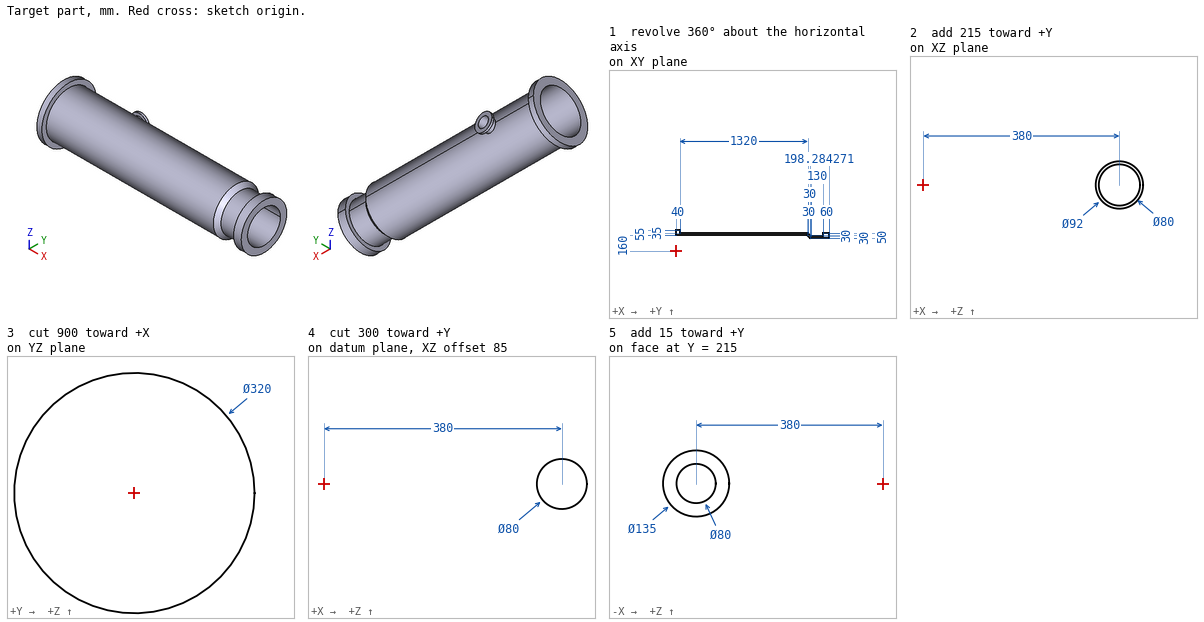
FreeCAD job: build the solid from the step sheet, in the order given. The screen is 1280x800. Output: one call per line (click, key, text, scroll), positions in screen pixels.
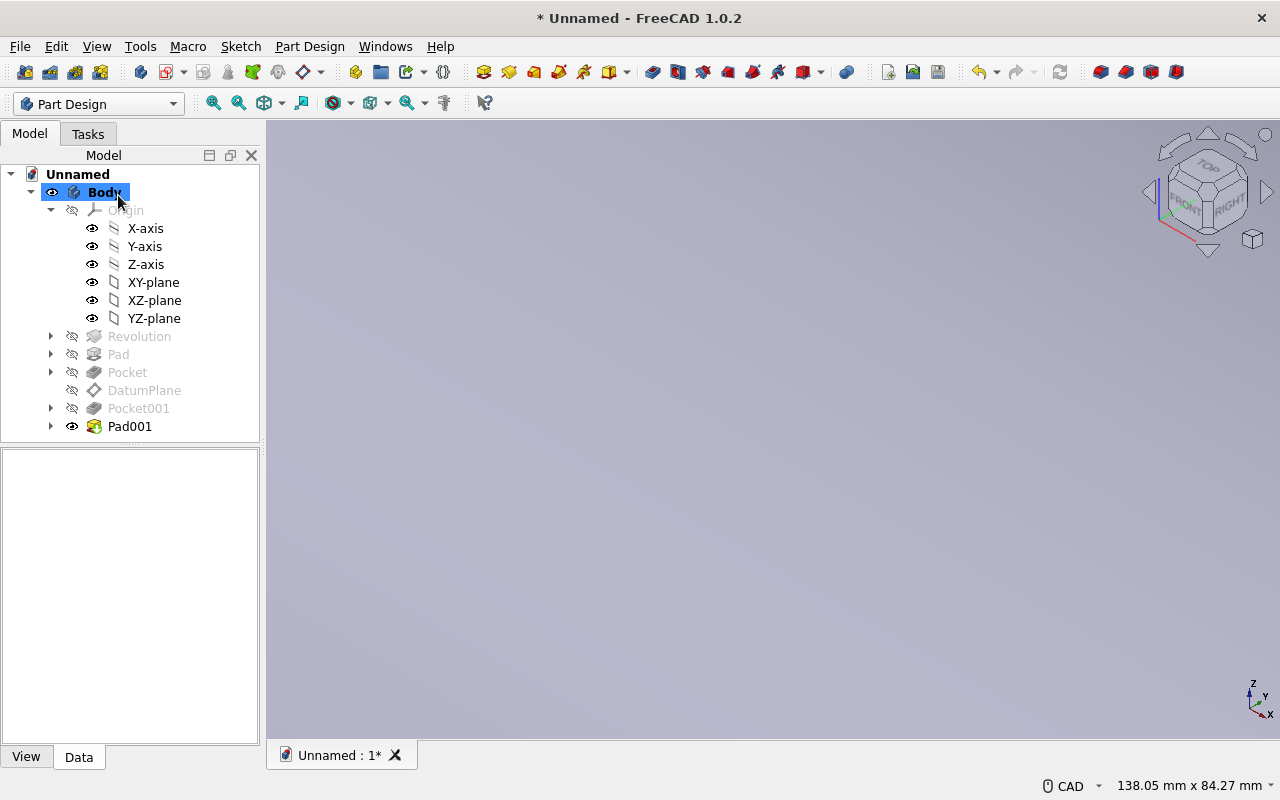
key(v)
key(f)